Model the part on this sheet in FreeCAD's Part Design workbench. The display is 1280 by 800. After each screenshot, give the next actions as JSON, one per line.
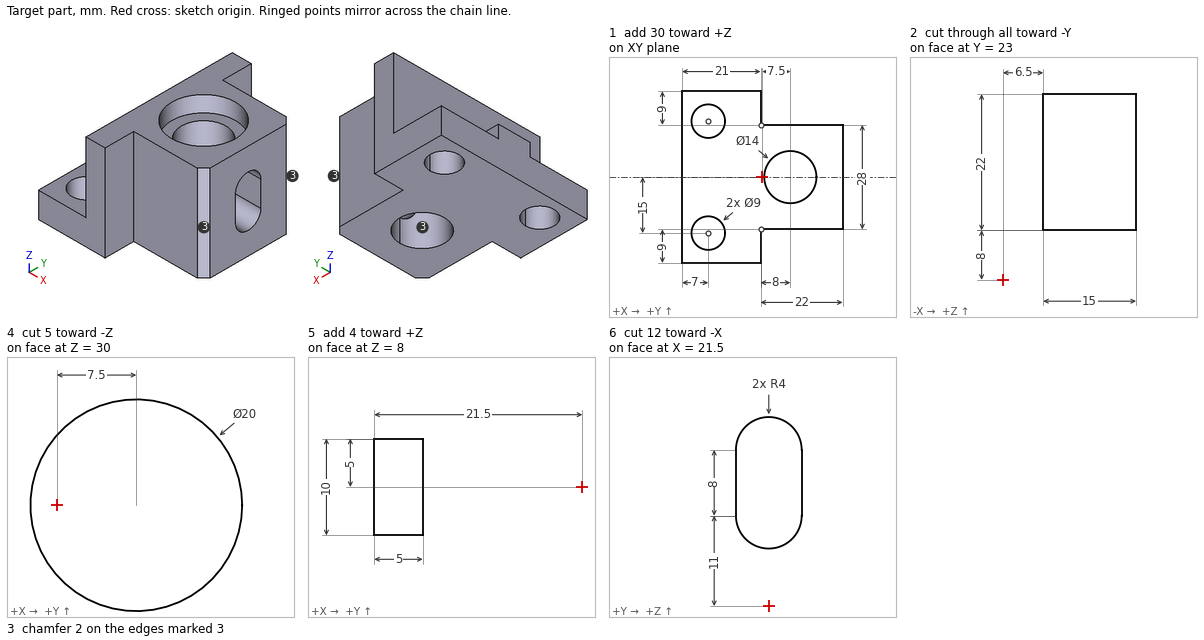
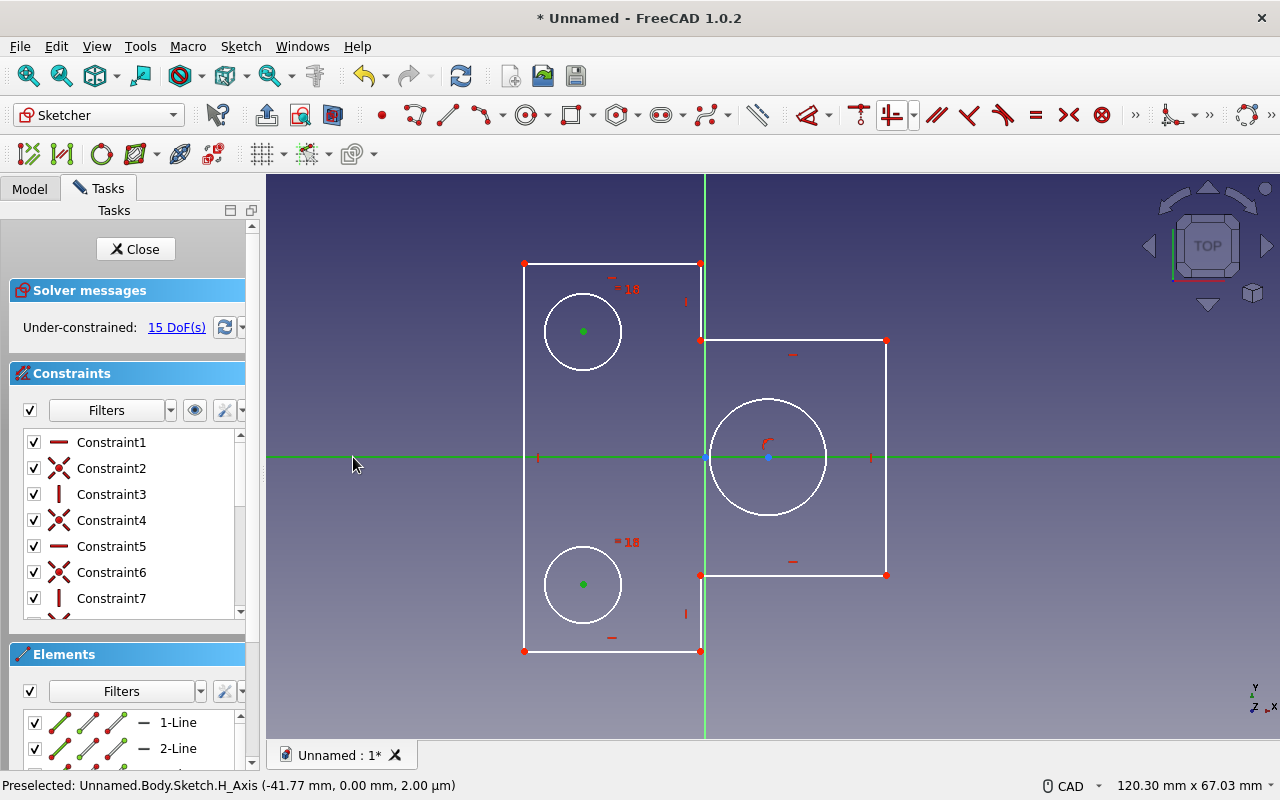
{"action": "key", "text": "s"}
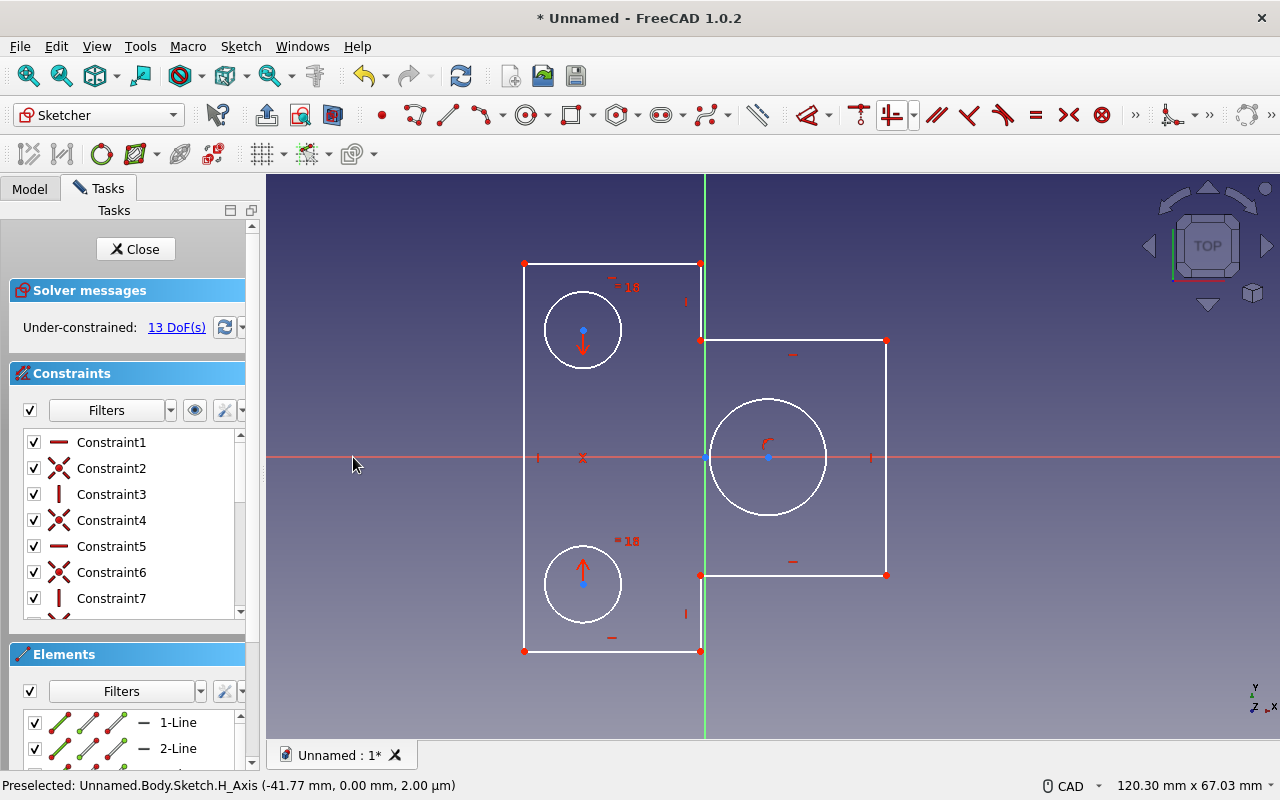
{"action": "left_click", "coordinate": [701, 576]}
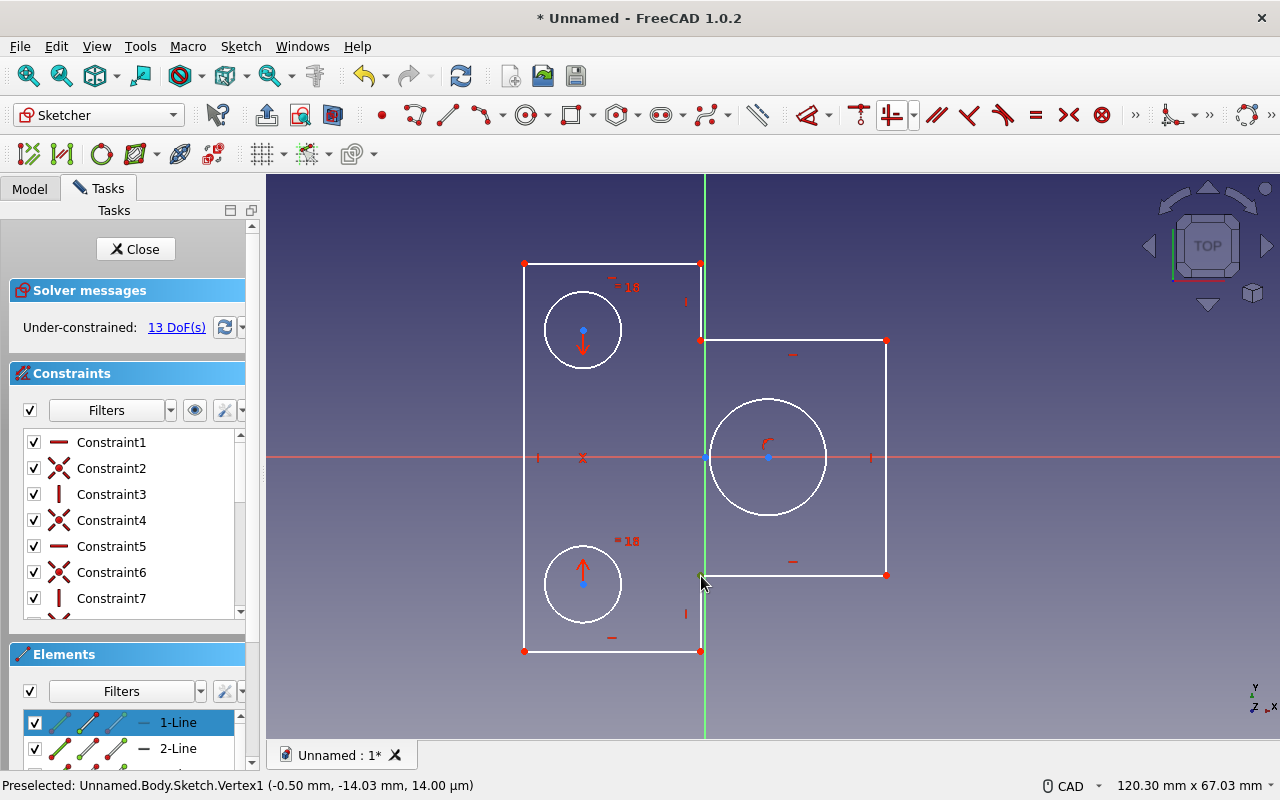
{"action": "left_click", "coordinate": [701, 340]}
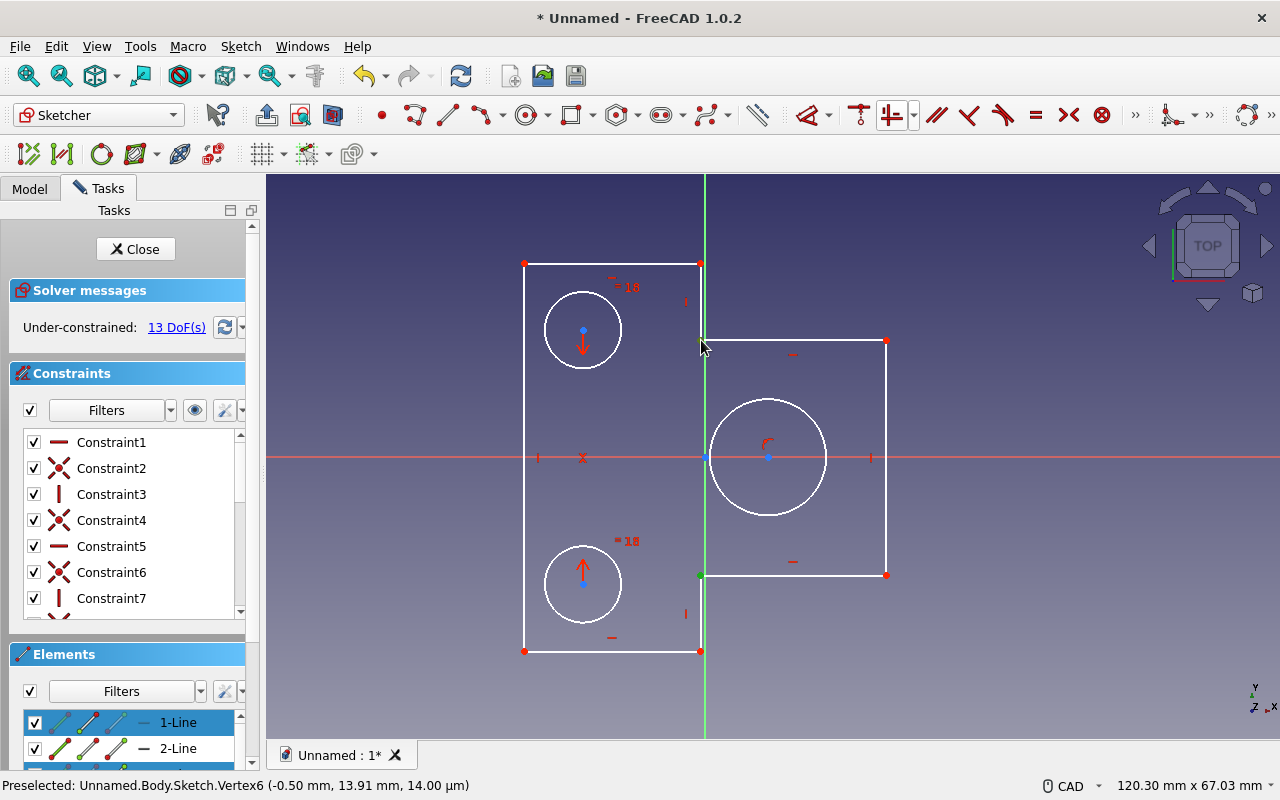
{"action": "left_click", "coordinate": [353, 457]}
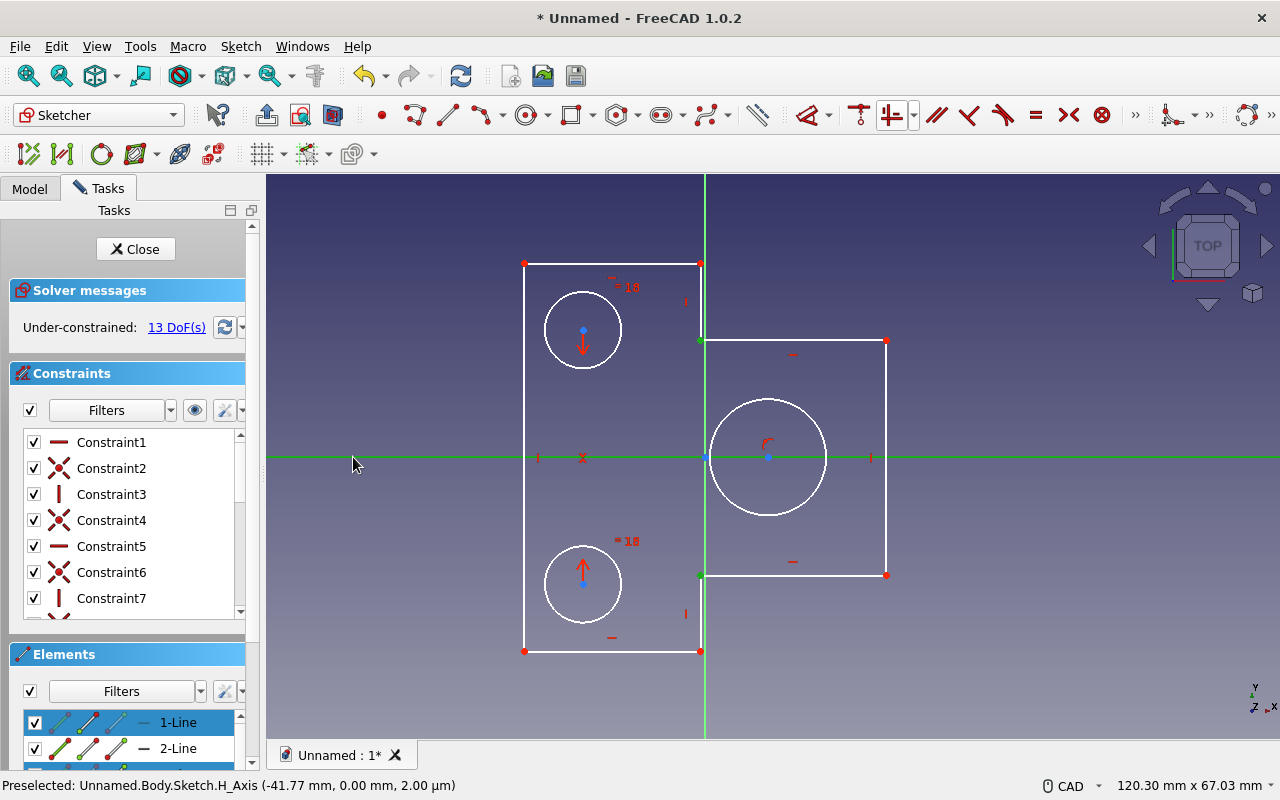
{"action": "left_click", "coordinate": [1069, 116]}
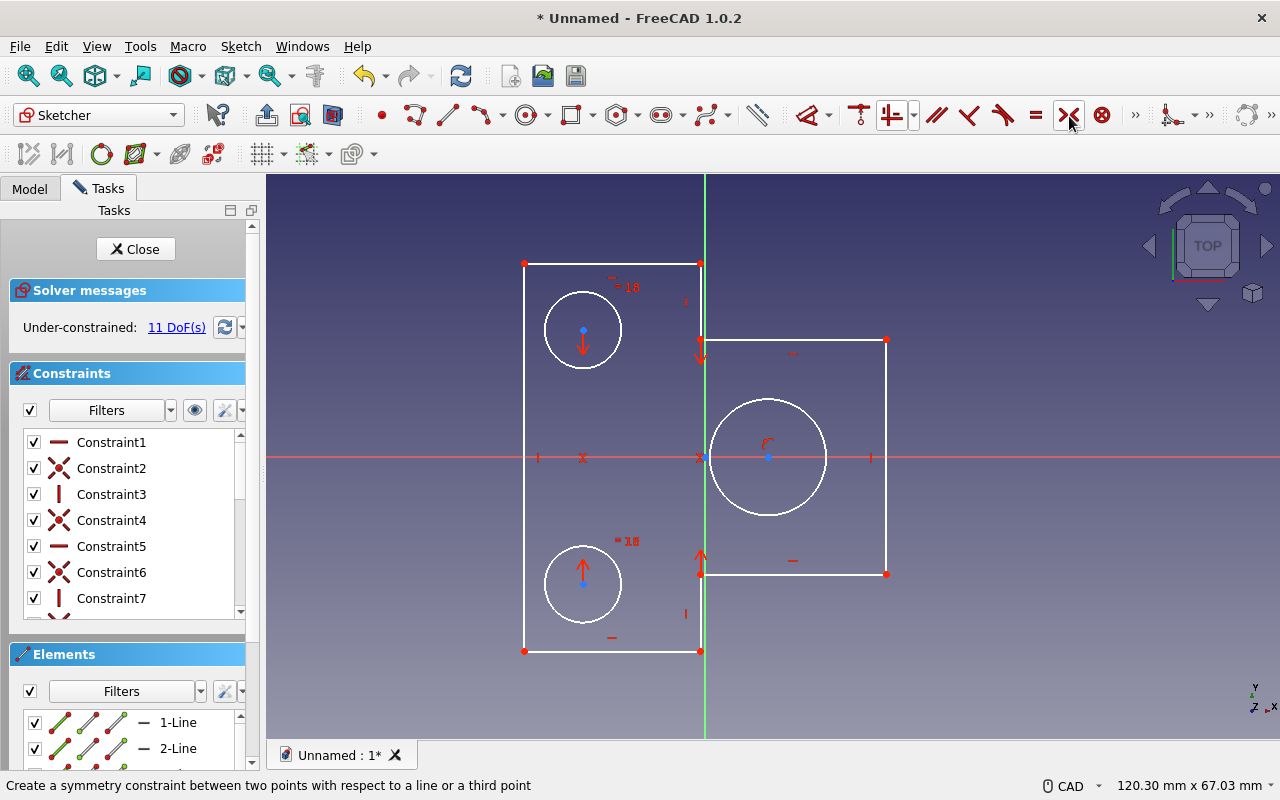
{"action": "key", "text": "d"}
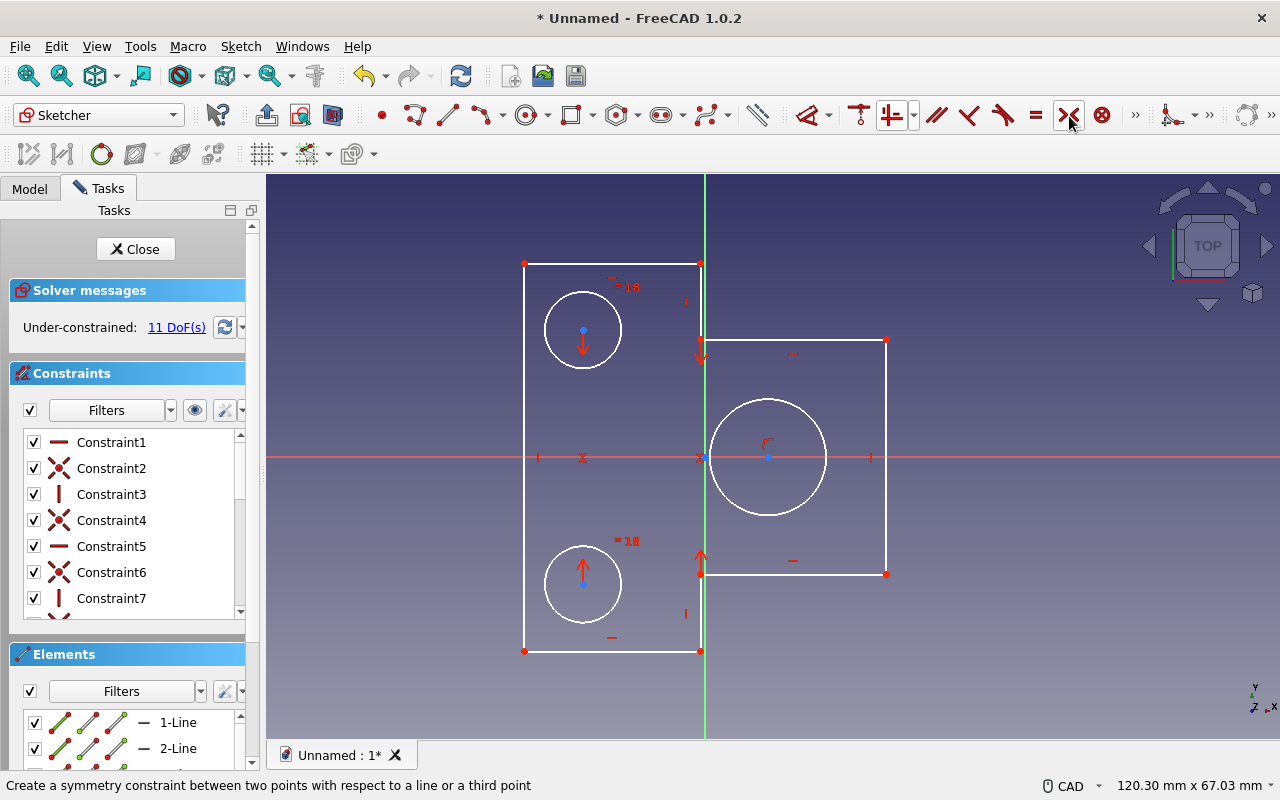
{"action": "left_click", "coordinate": [610, 557]}
{"action": "left_click", "coordinate": [632, 534]}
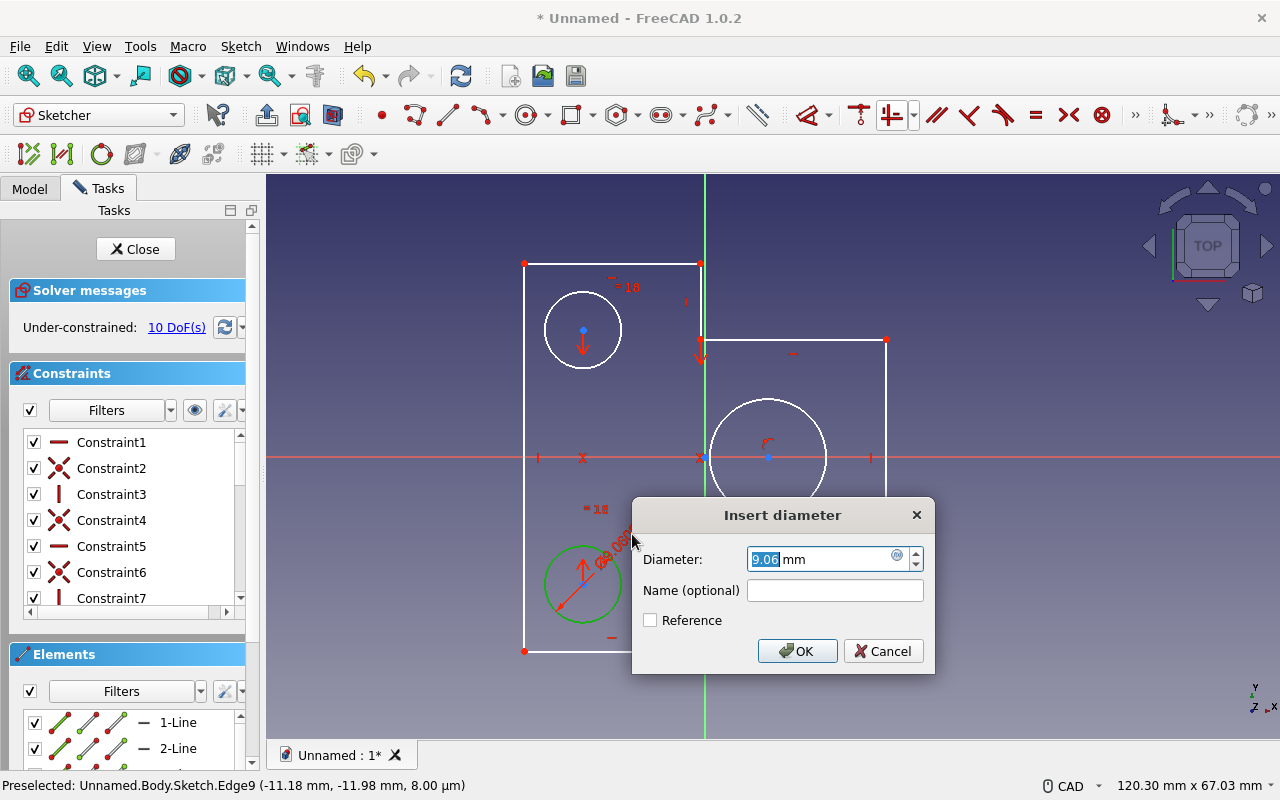
{"action": "type", "text": "9"}
{"action": "key", "text": "Return"}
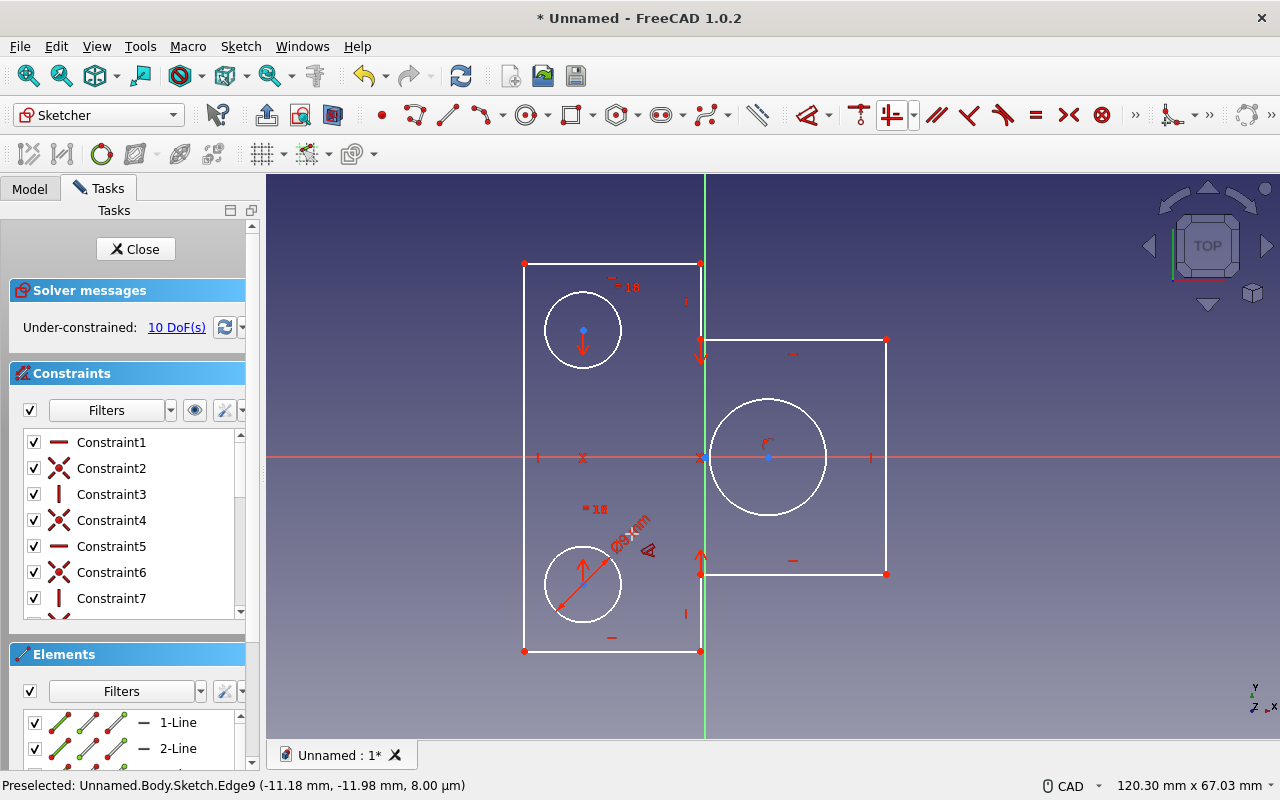
{"action": "left_click", "coordinate": [809, 416]}
{"action": "left_click", "coordinate": [832, 393]}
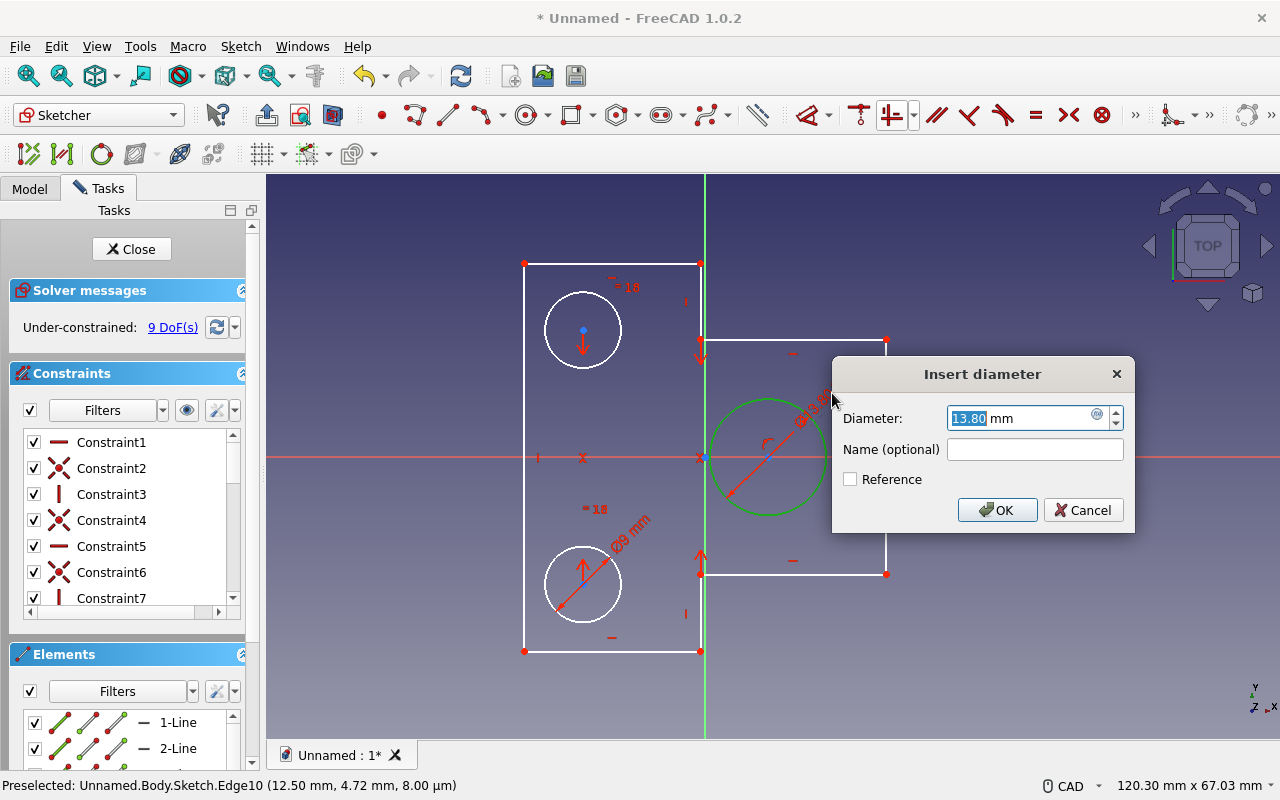
{"action": "type", "text": "14"}
{"action": "key", "text": "Return"}